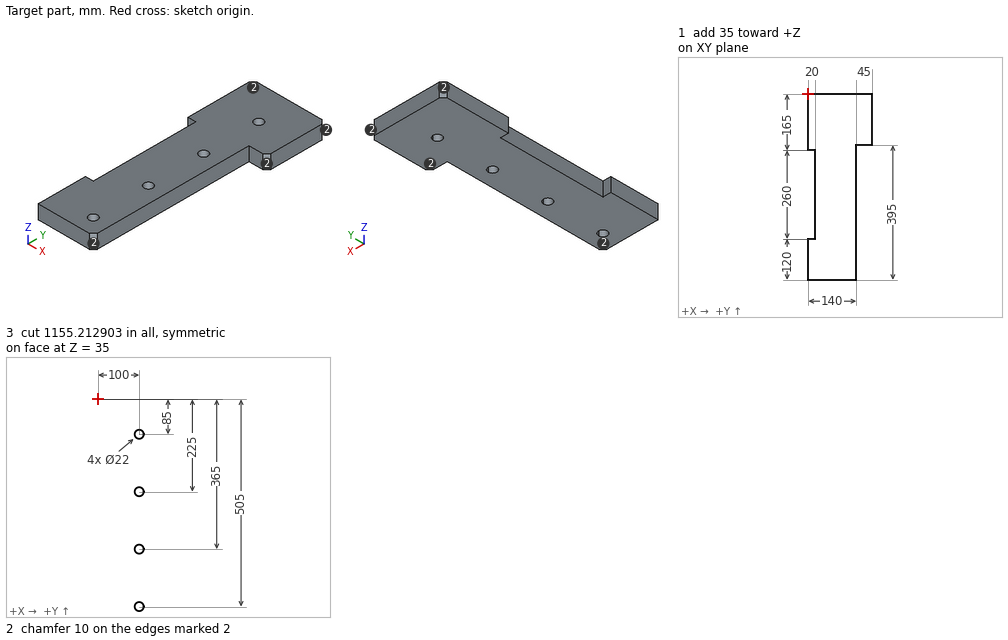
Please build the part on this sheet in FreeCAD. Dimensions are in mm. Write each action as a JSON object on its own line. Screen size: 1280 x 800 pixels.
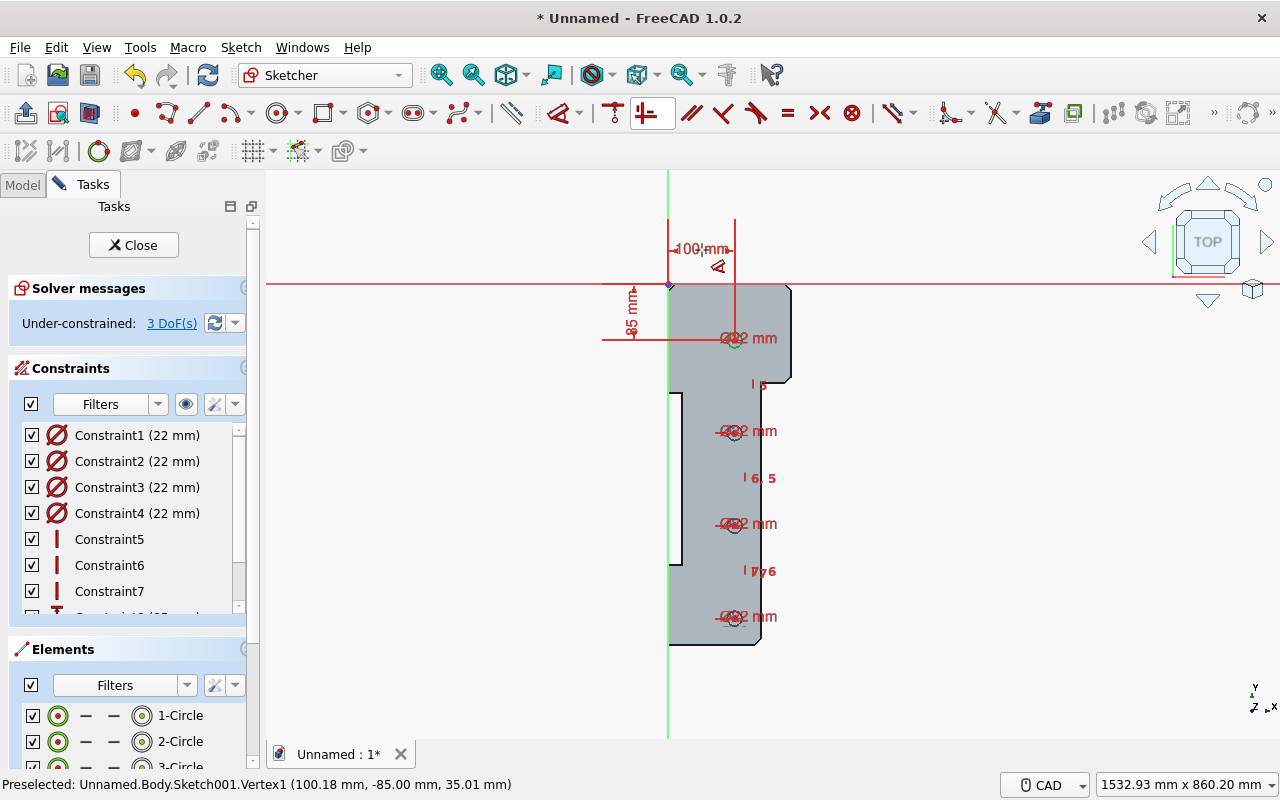
{"action": "left_click", "coordinate": [735, 433]}
{"action": "left_click", "coordinate": [634, 359]}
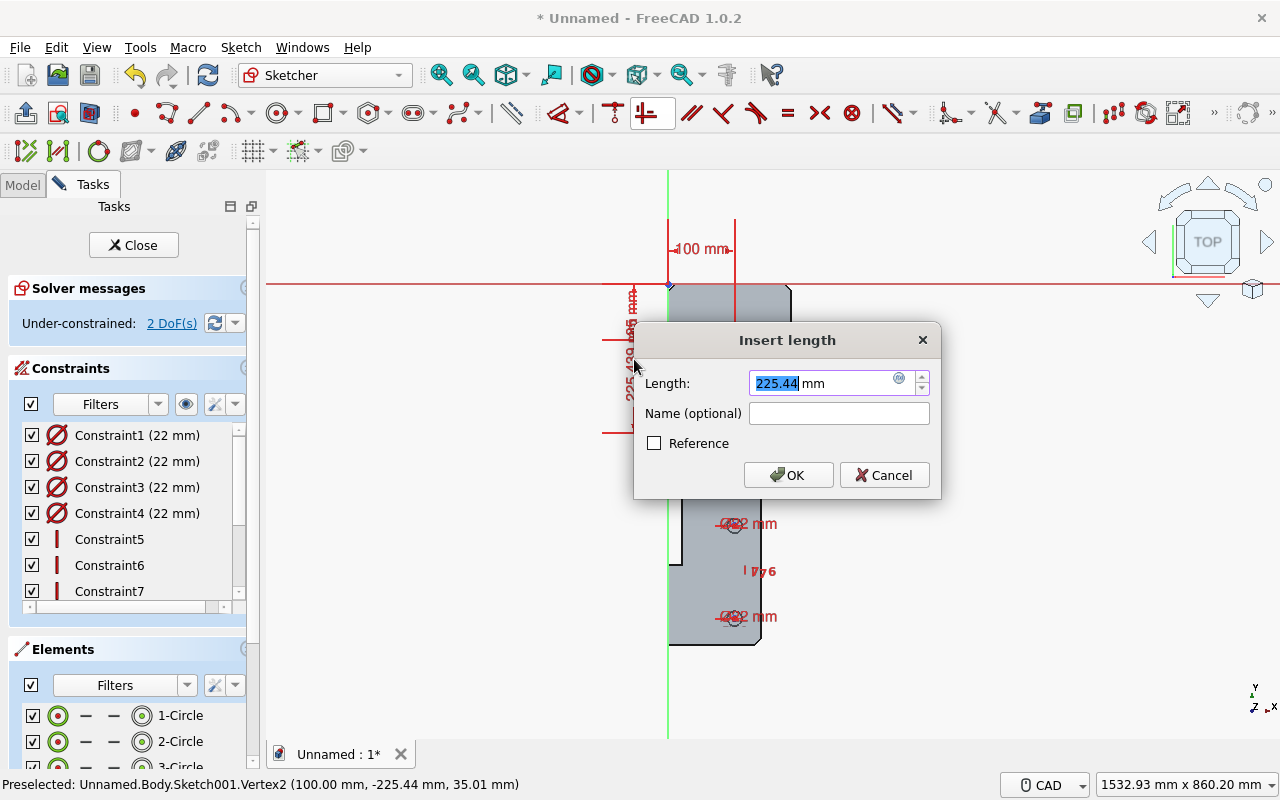
{"action": "type", "text": "225"}
{"action": "key", "text": "Return"}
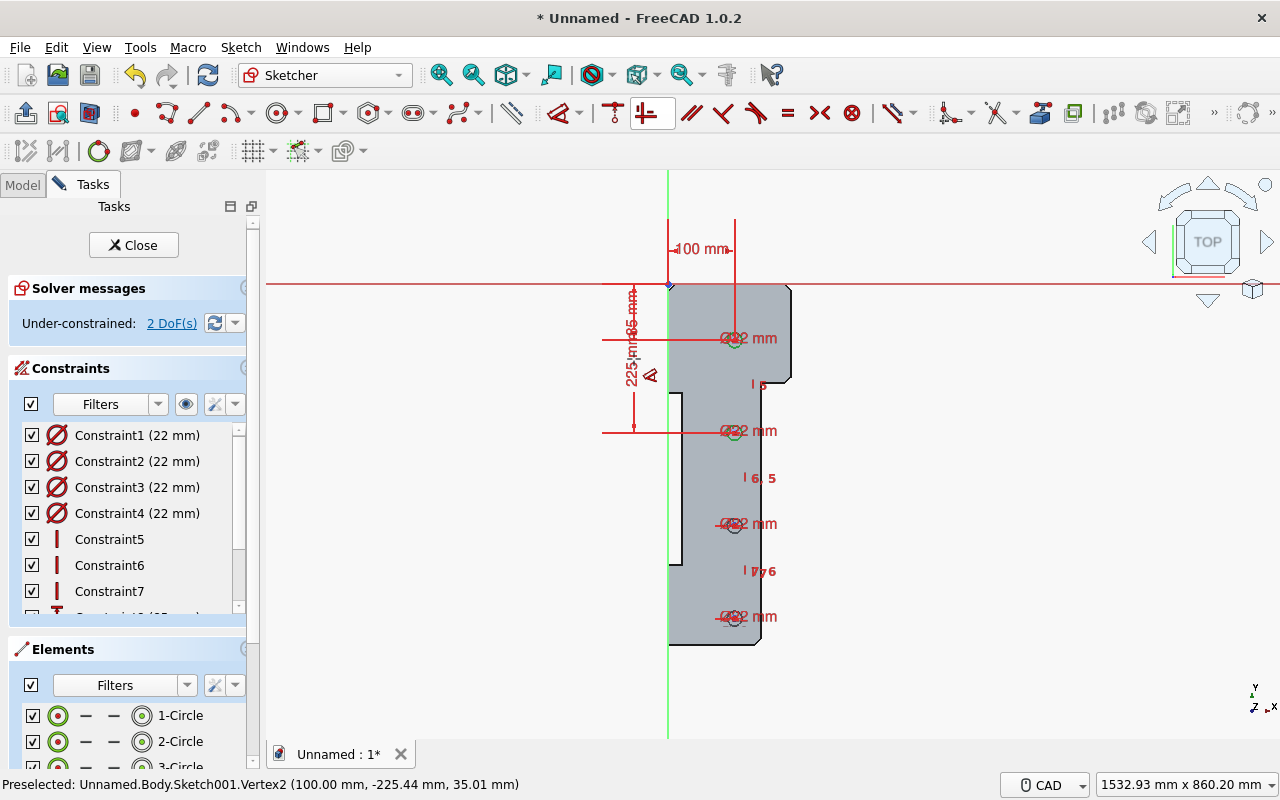
{"action": "left_click", "coordinate": [735, 526]}
{"action": "left_click", "coordinate": [634, 405]}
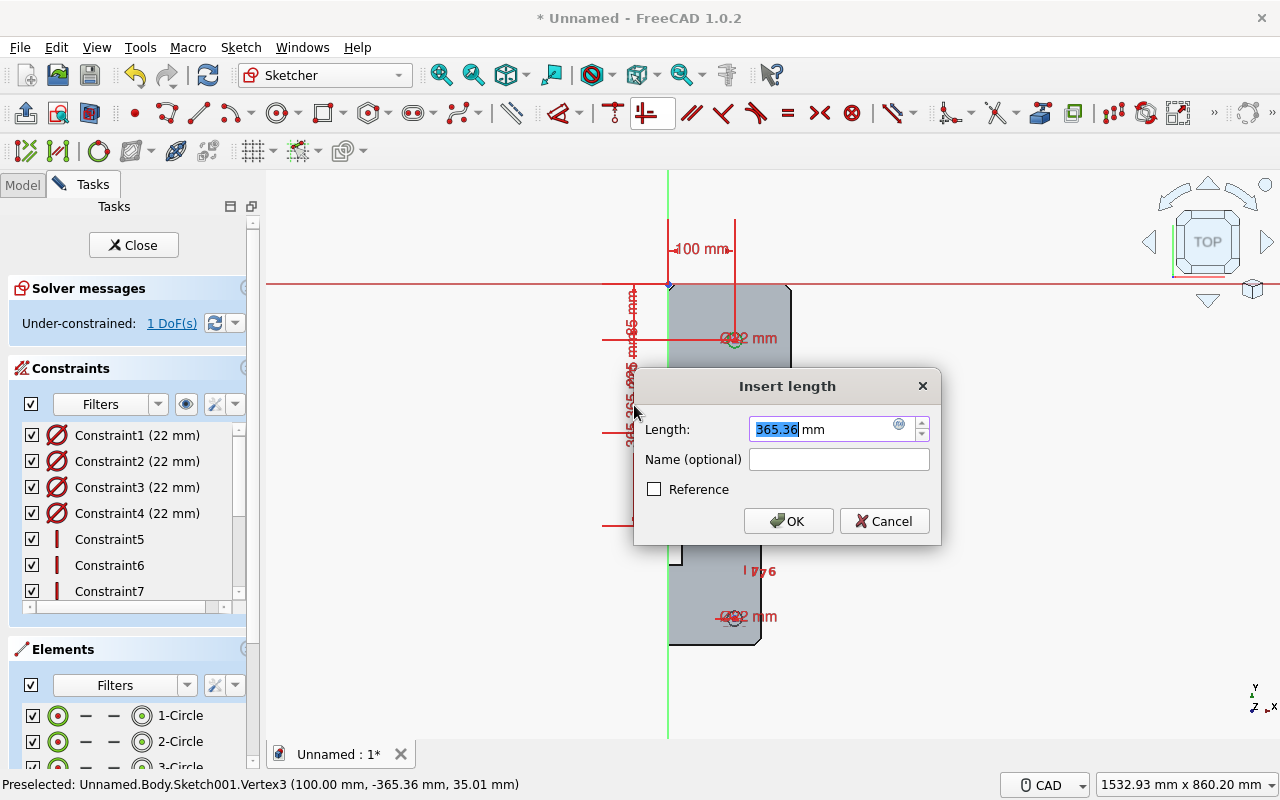
{"action": "type", "text": "365"}
{"action": "key", "text": "Return"}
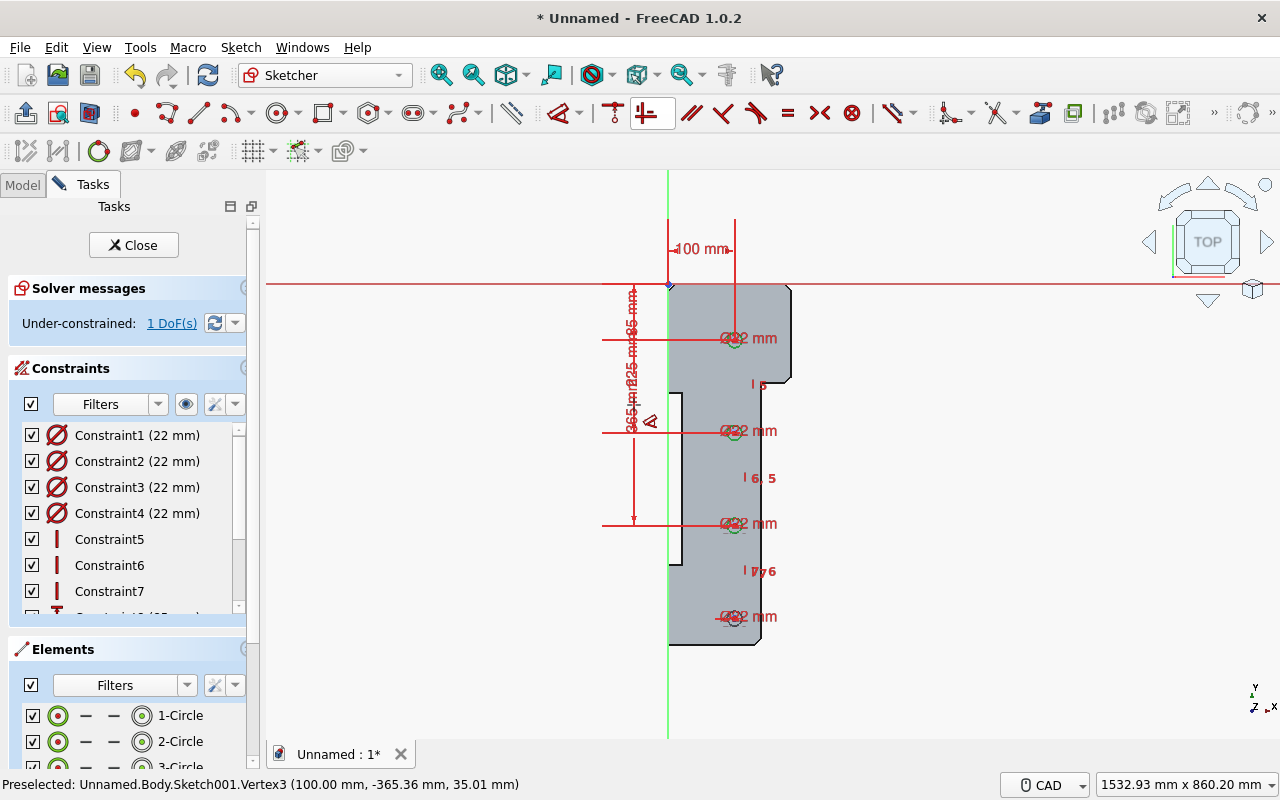
{"action": "left_click", "coordinate": [735, 619]}
{"action": "left_click", "coordinate": [634, 451]}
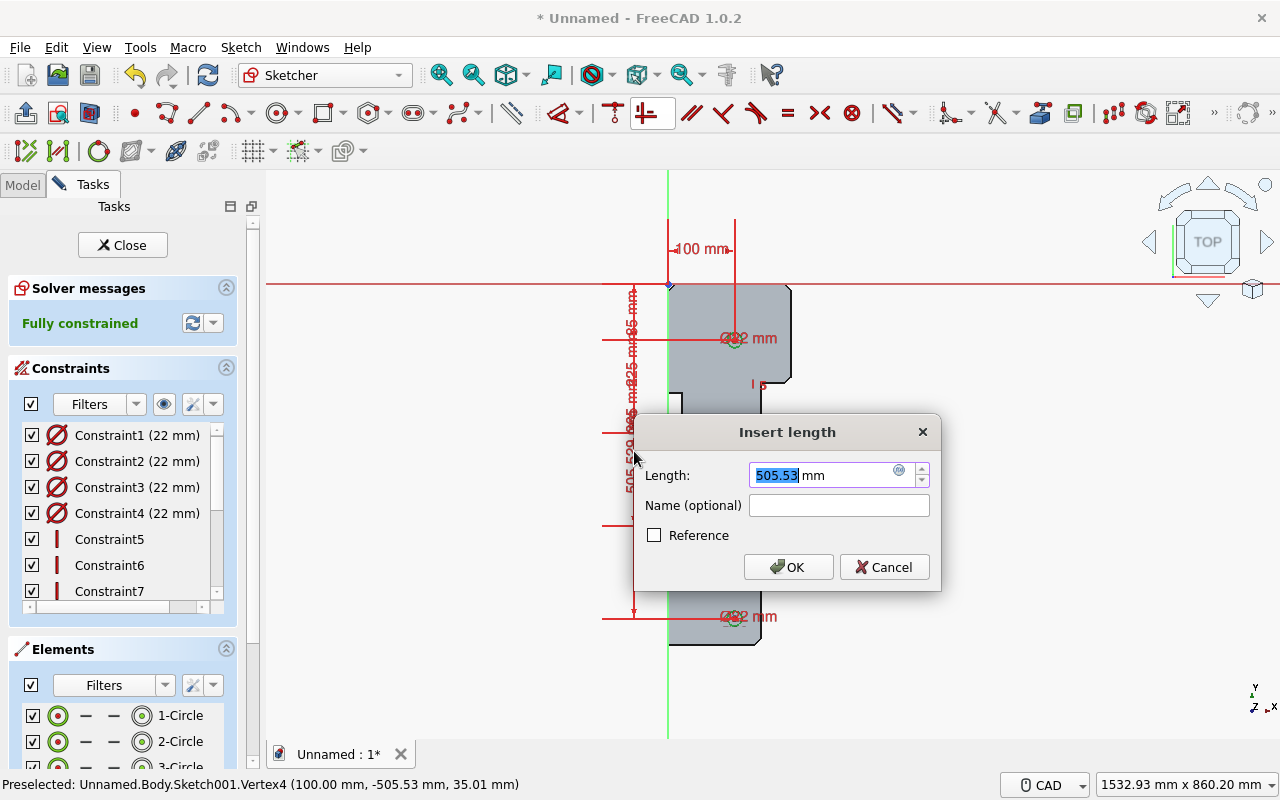
{"action": "type", "text": "505"}
{"action": "key", "text": "Return"}
{"action": "key", "text": "Escape"}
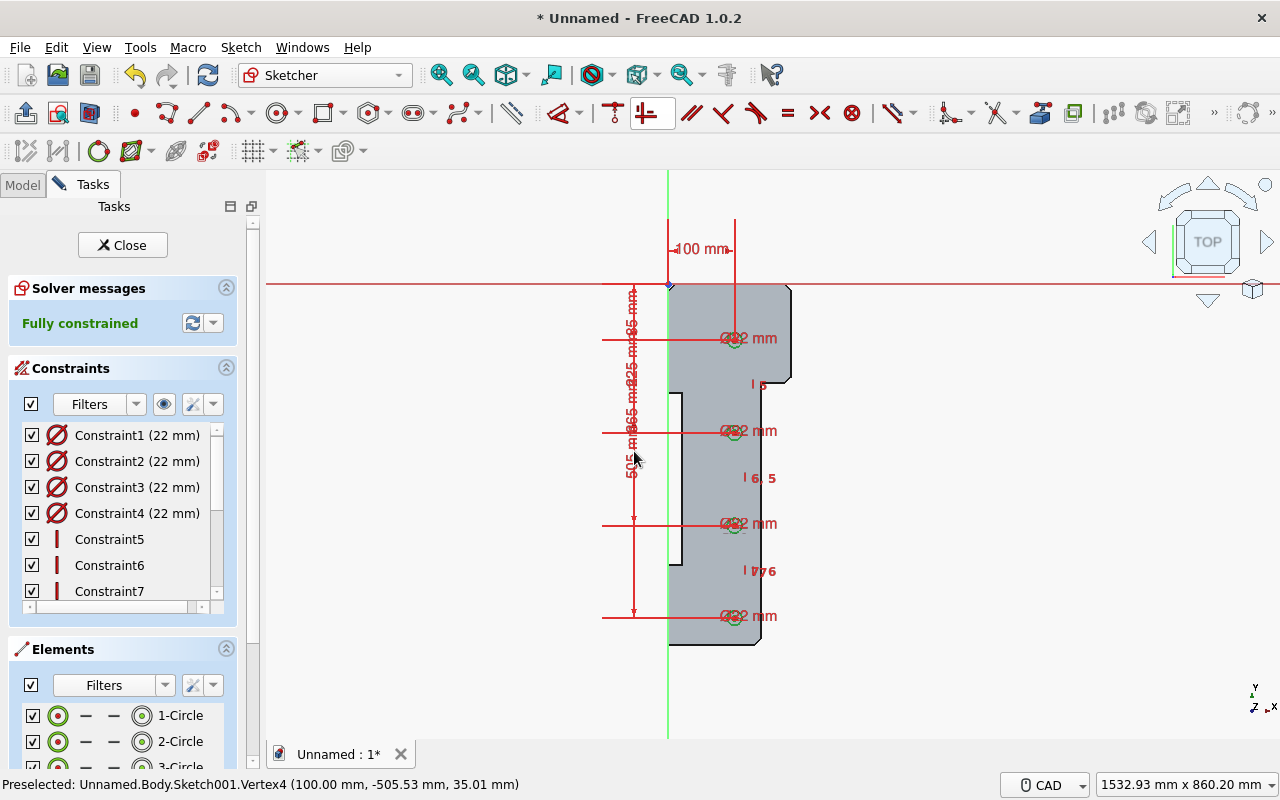
{"action": "left_click", "coordinate": [123, 245]}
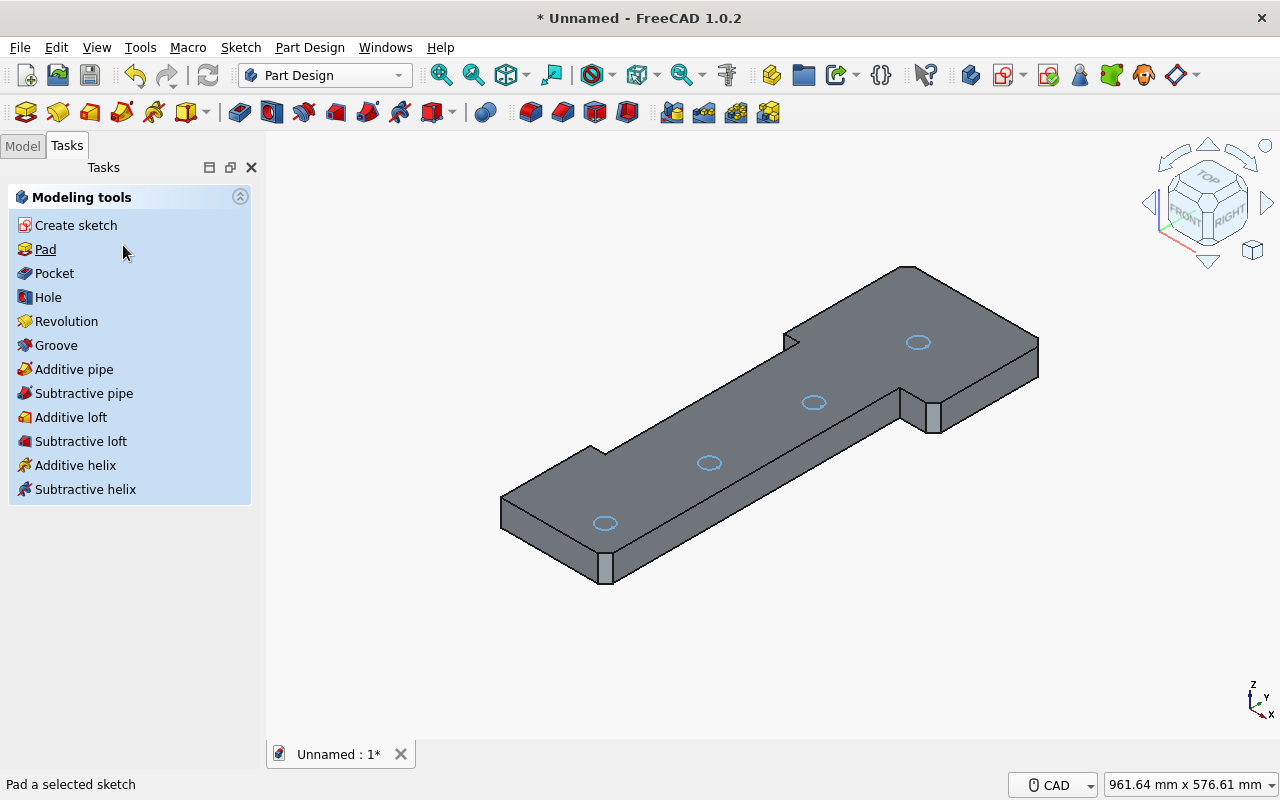
{"action": "left_click", "coordinate": [240, 112]}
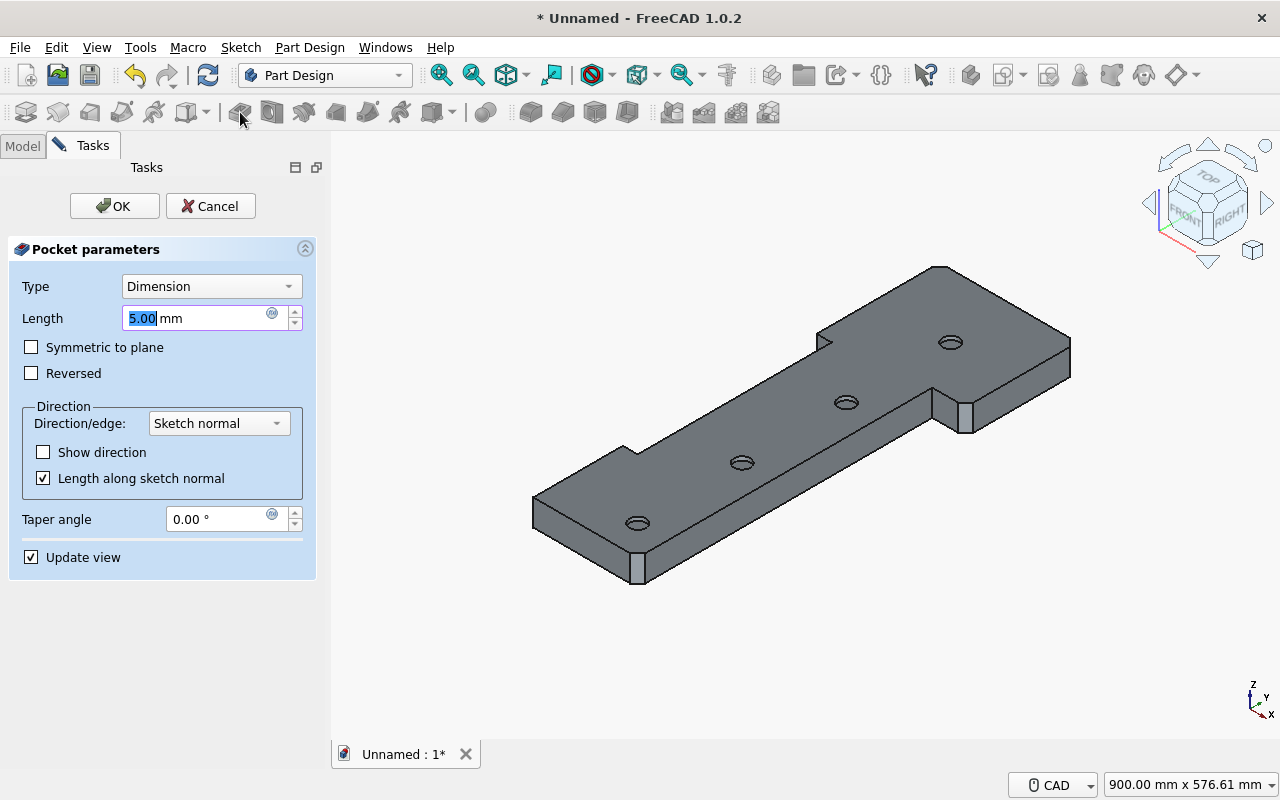
{"action": "type", "text": "1155.212903"}
{"action": "key", "text": "Tab"}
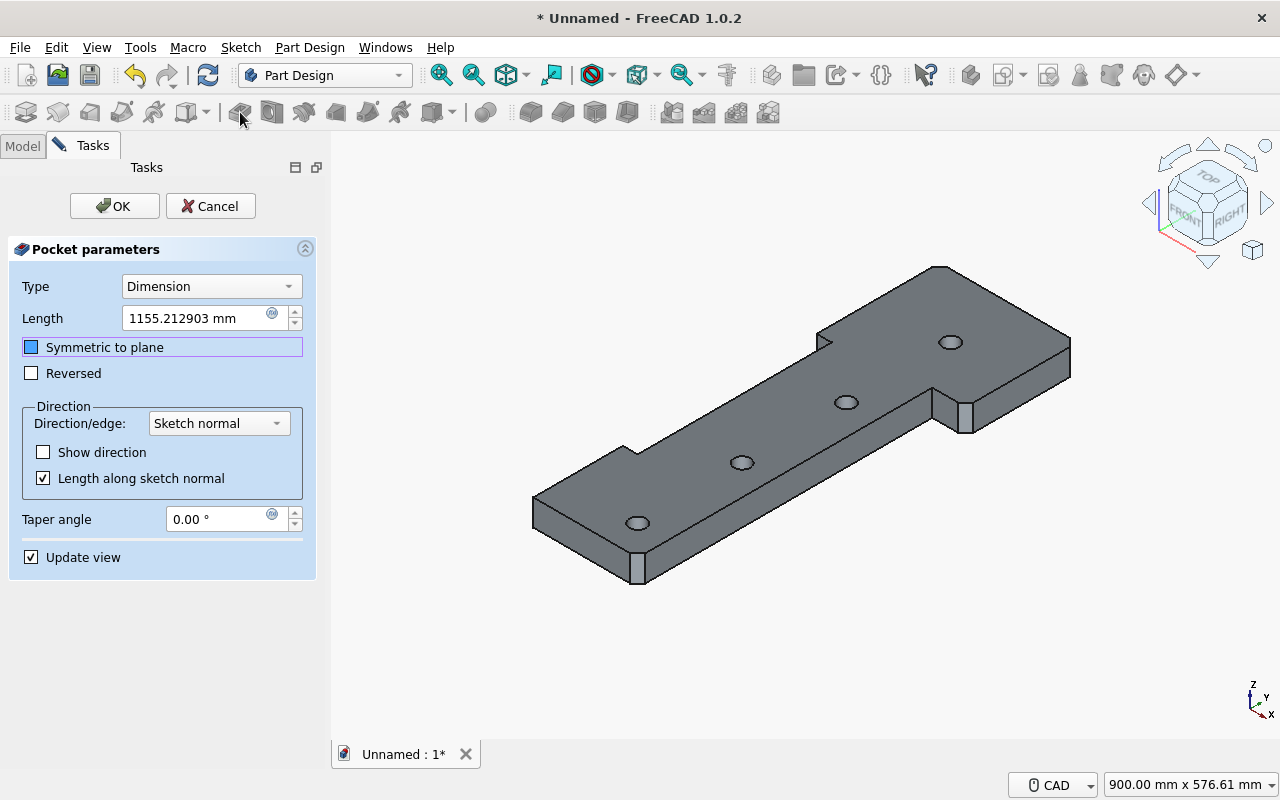
{"action": "left_click", "coordinate": [30, 347]}